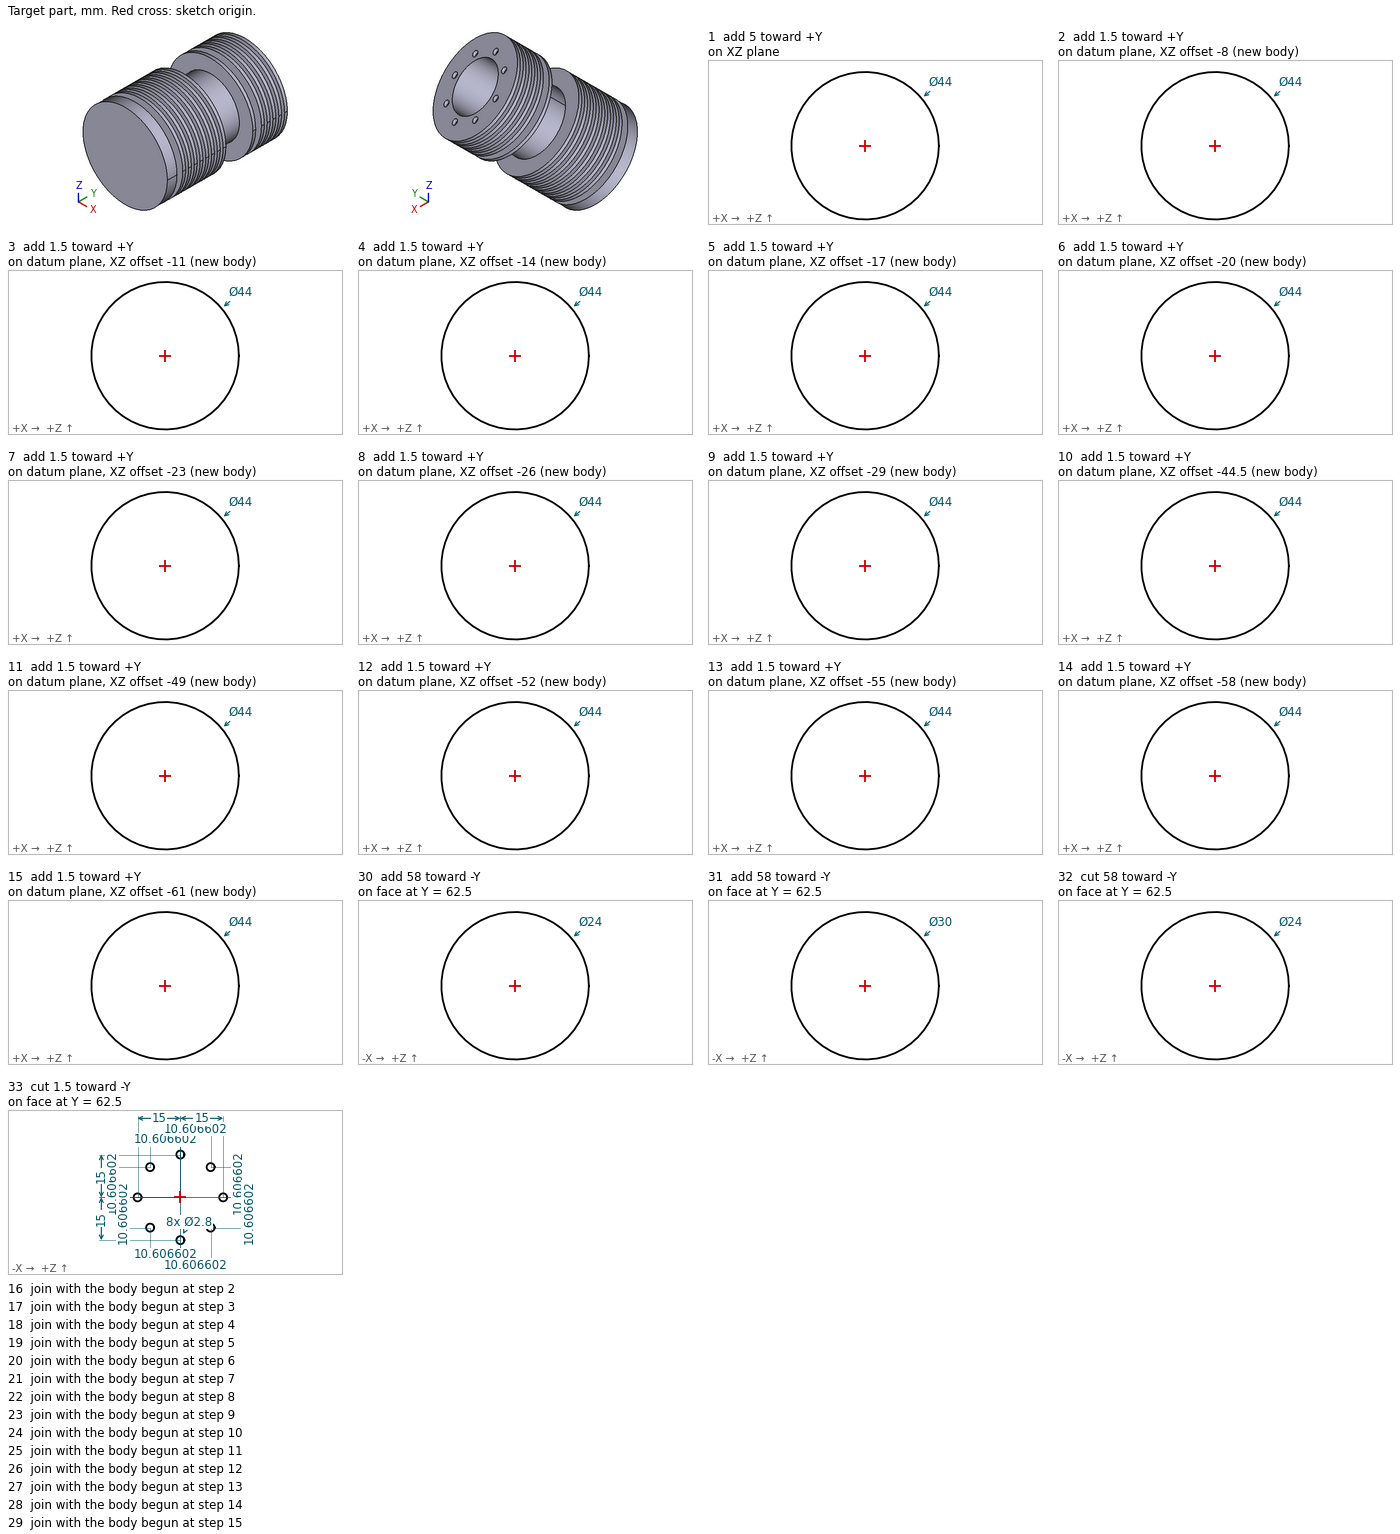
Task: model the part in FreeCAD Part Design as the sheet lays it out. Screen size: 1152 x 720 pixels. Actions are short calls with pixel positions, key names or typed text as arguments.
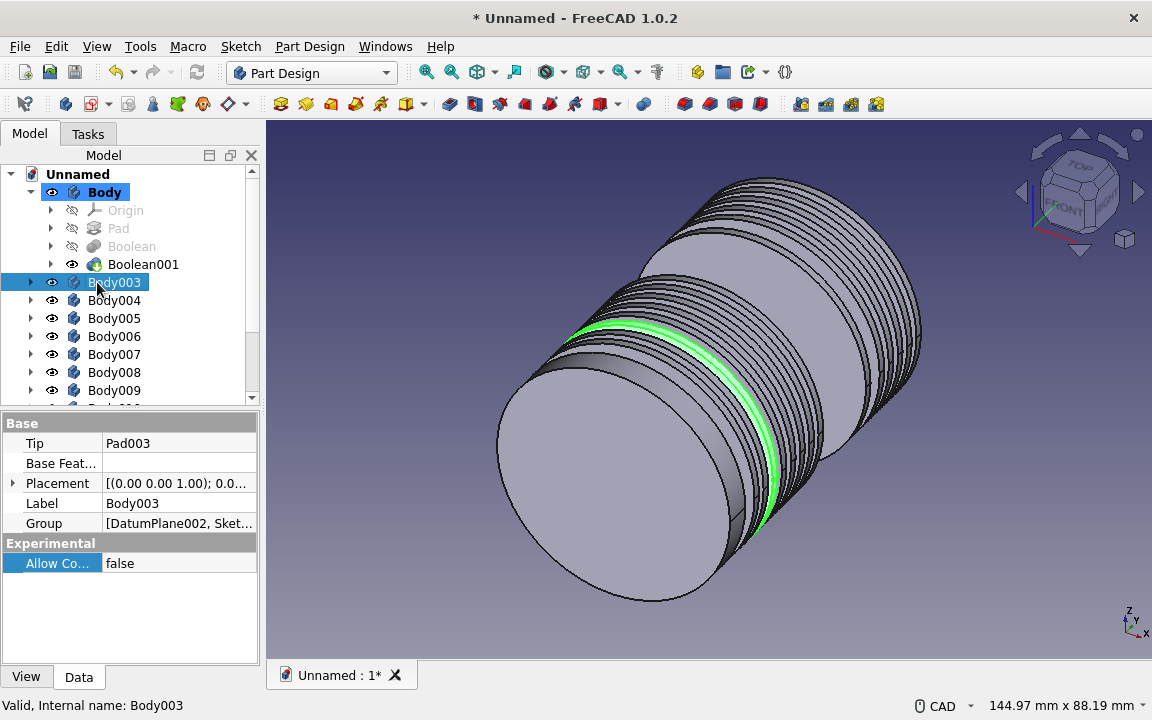
click(644, 104)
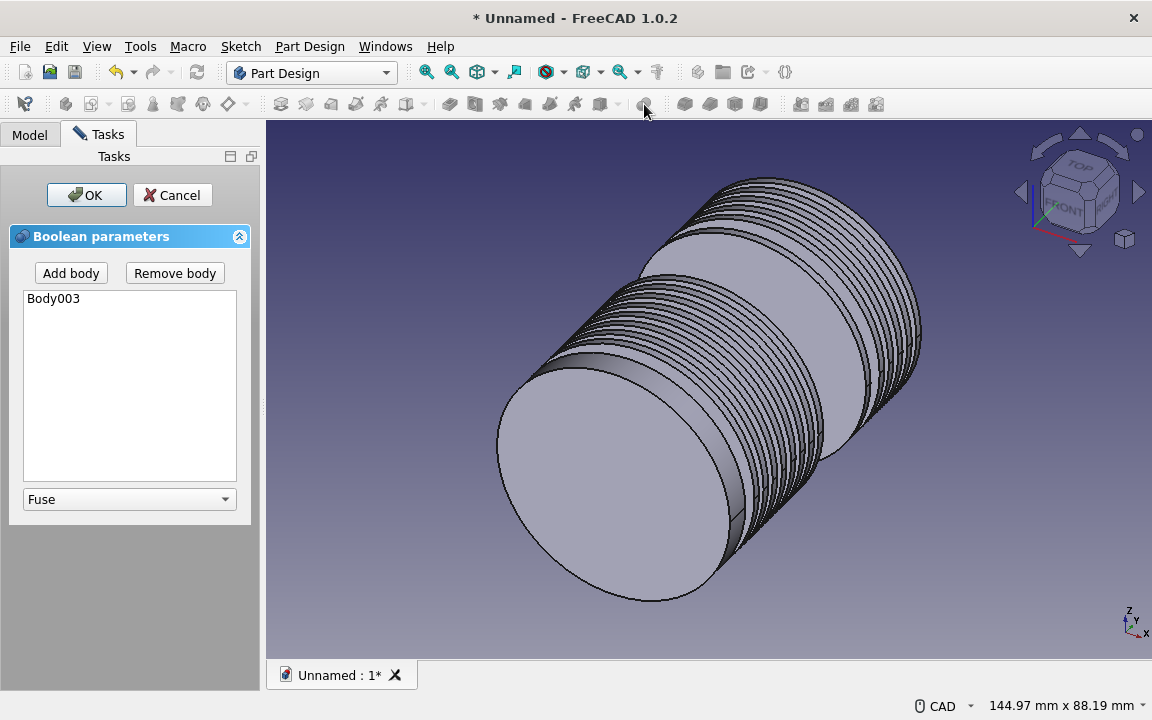
click(87, 195)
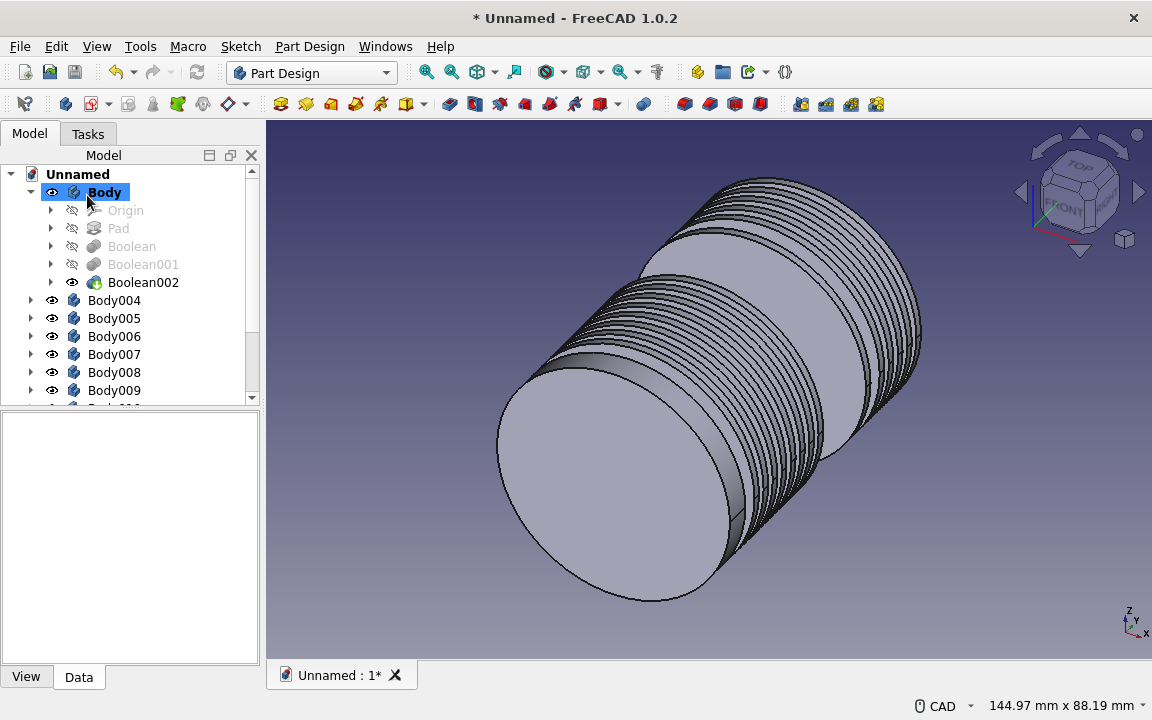
click(97, 300)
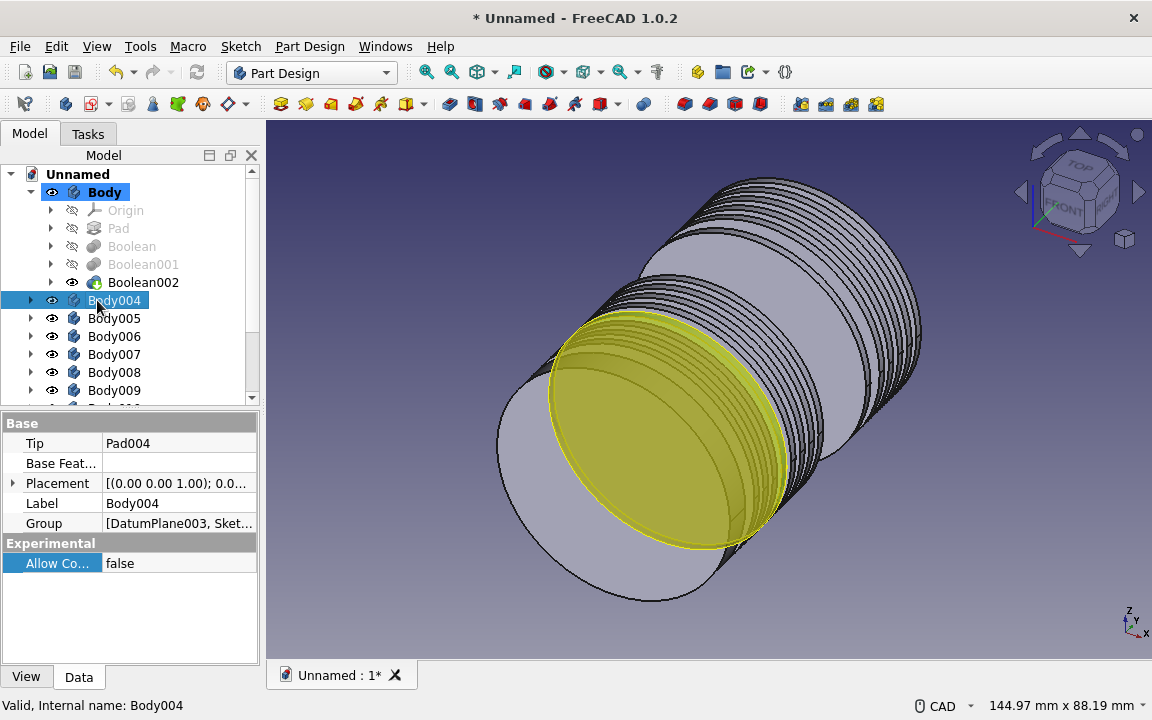
click(644, 104)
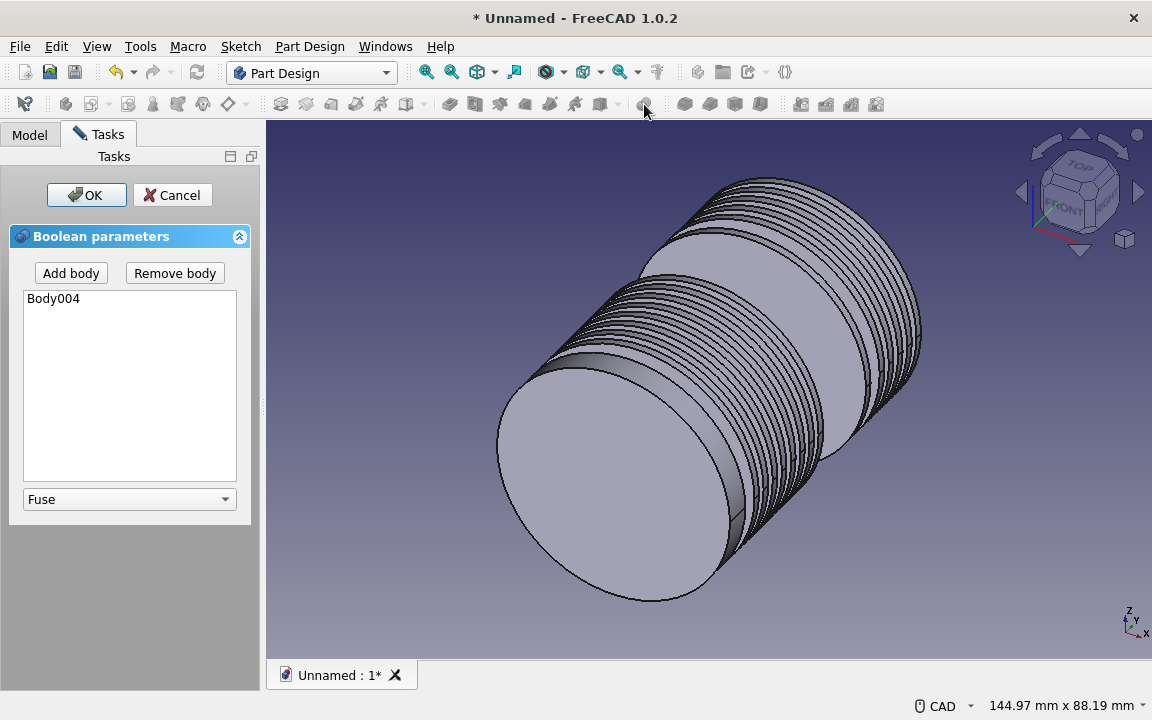
click(87, 195)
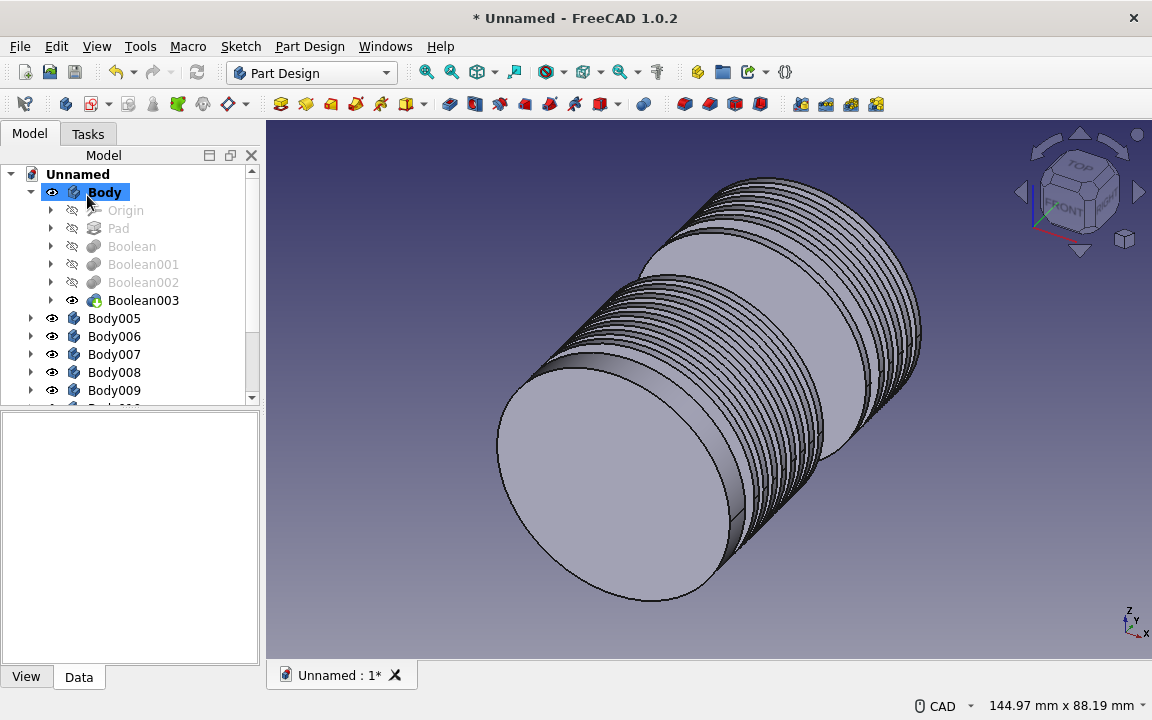
click(97, 318)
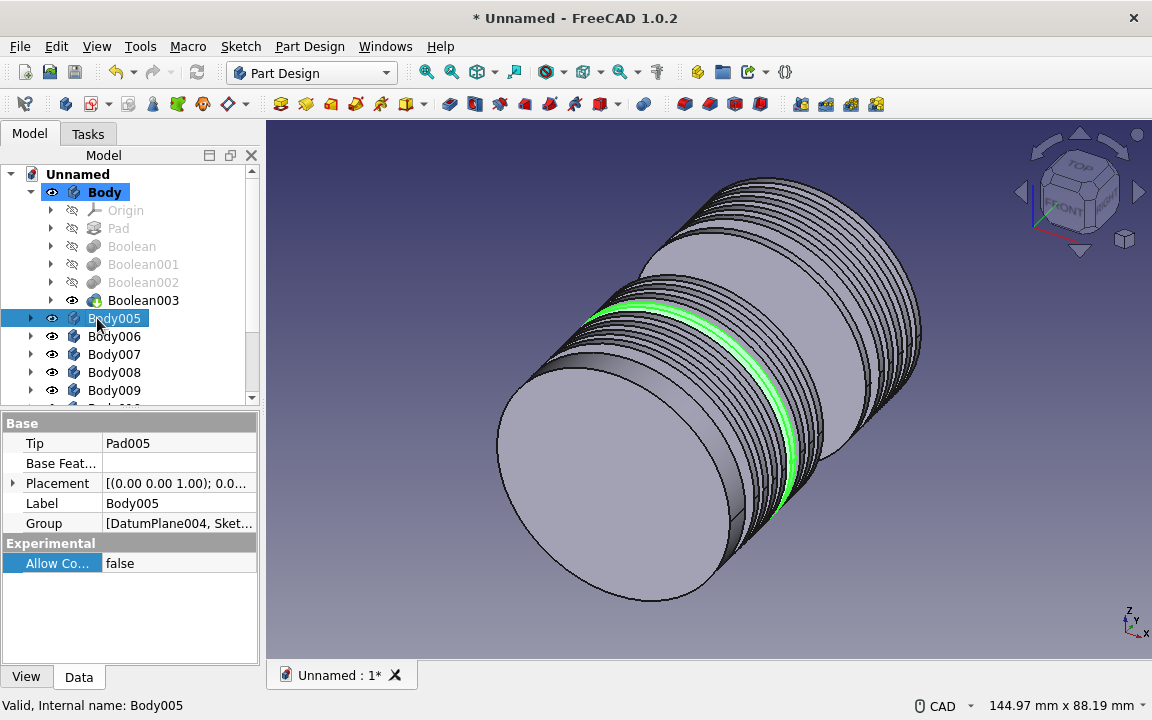
click(644, 104)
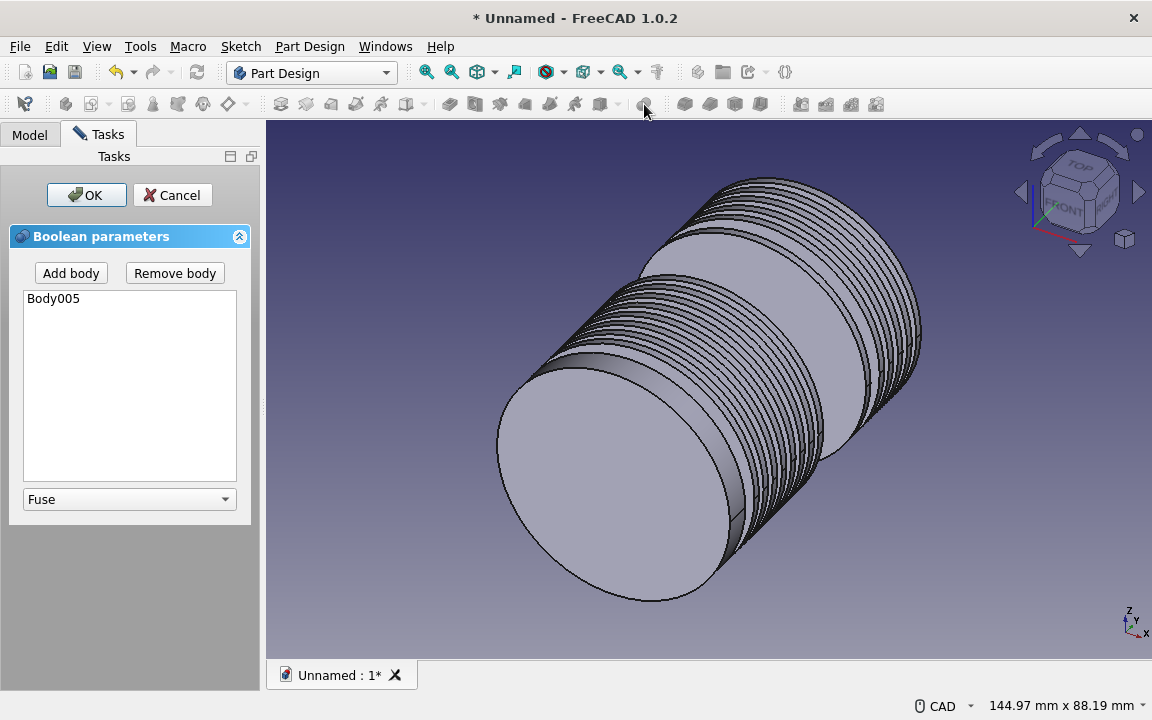
click(87, 195)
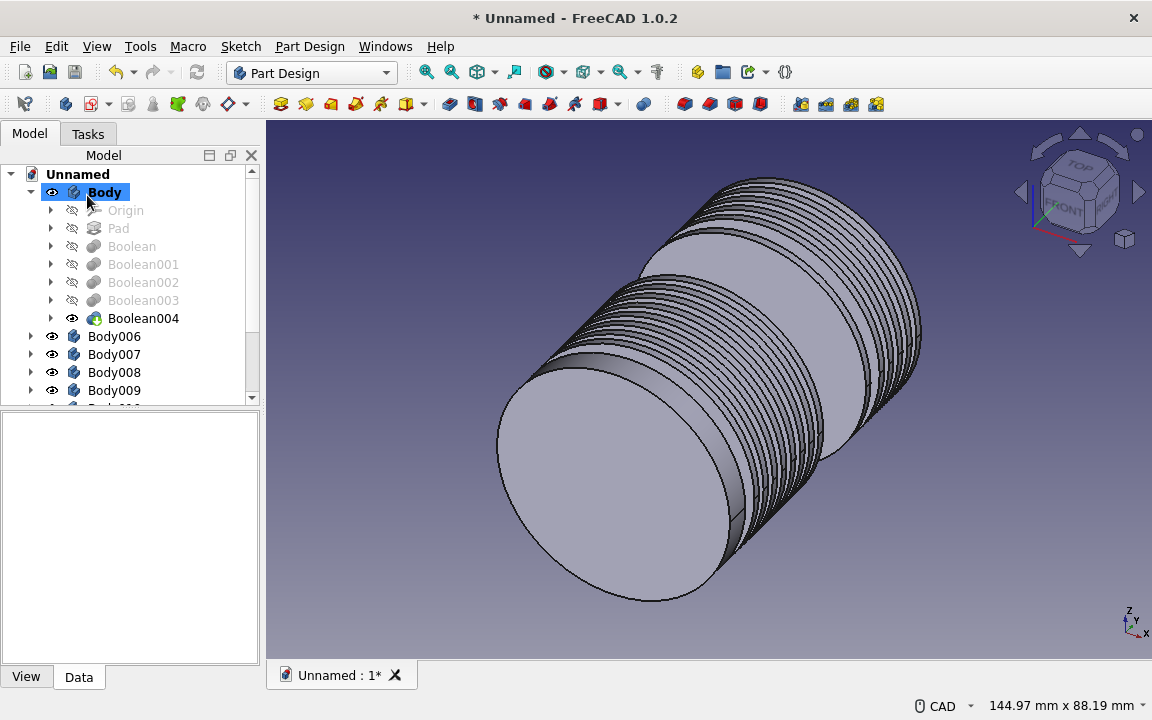
click(97, 336)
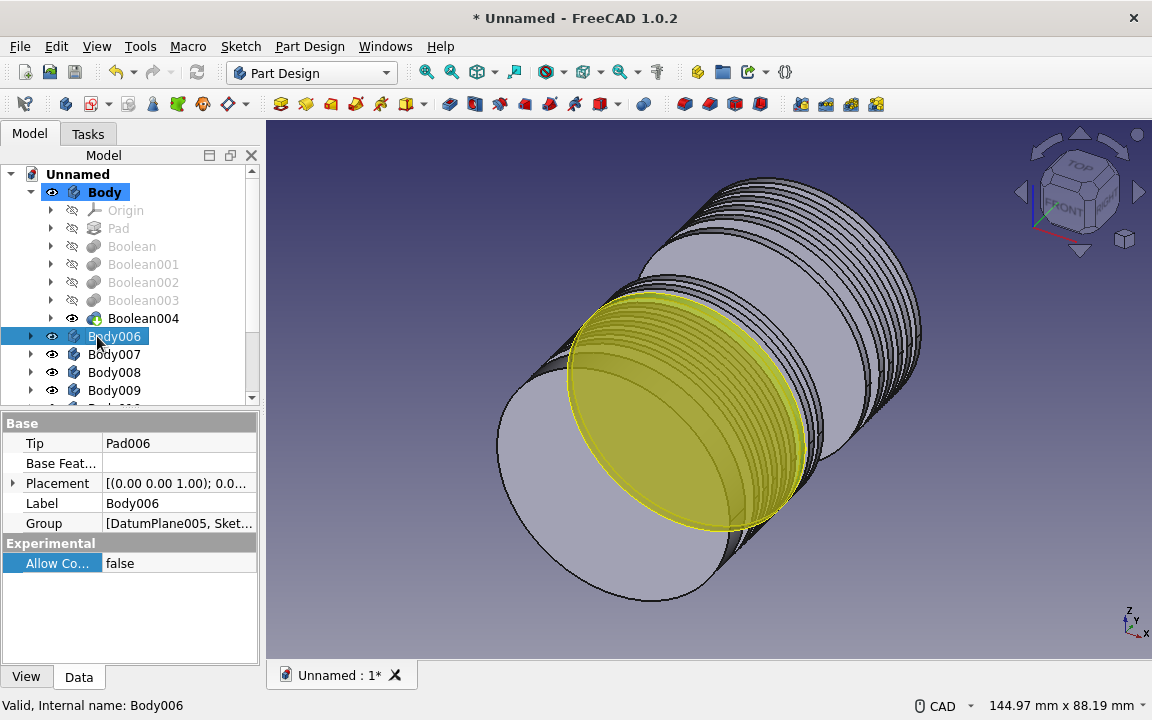
click(644, 104)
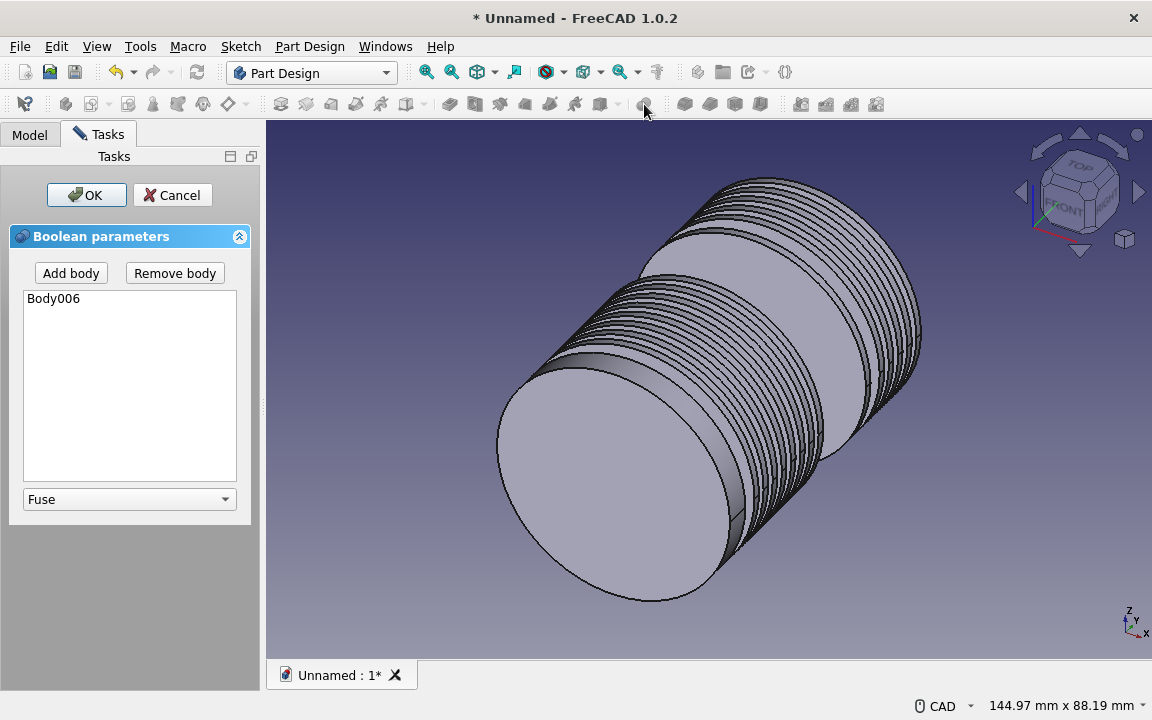
click(87, 195)